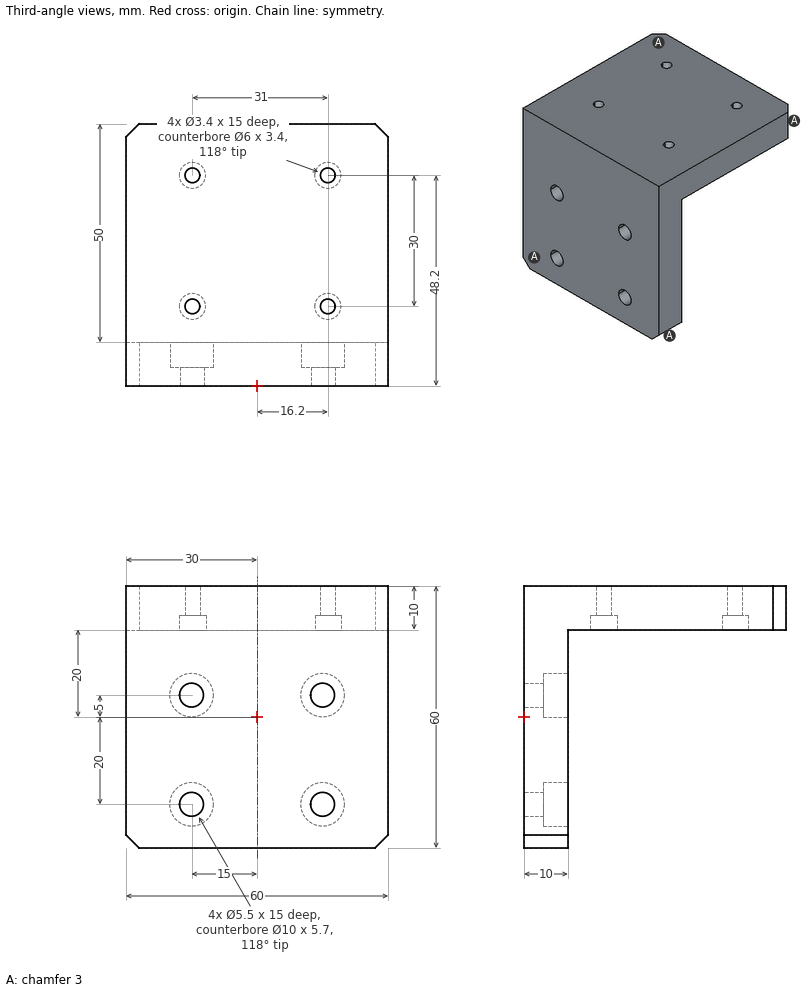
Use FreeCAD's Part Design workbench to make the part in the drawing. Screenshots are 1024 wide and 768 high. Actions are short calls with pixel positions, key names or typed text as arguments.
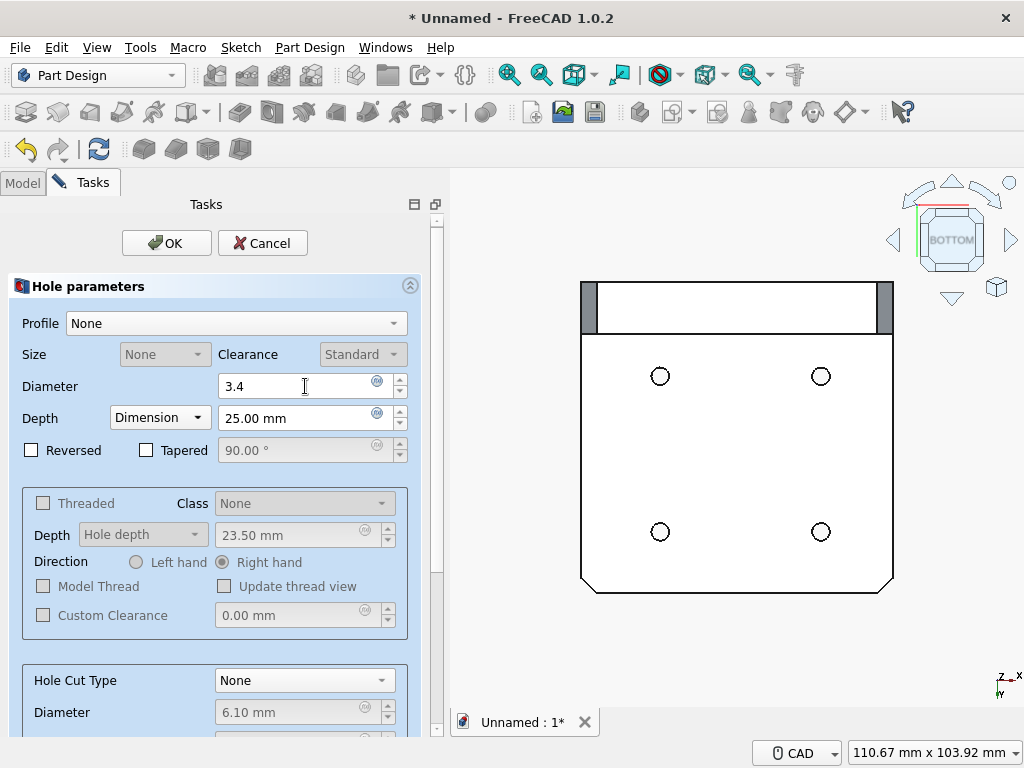
triple_click(305, 418)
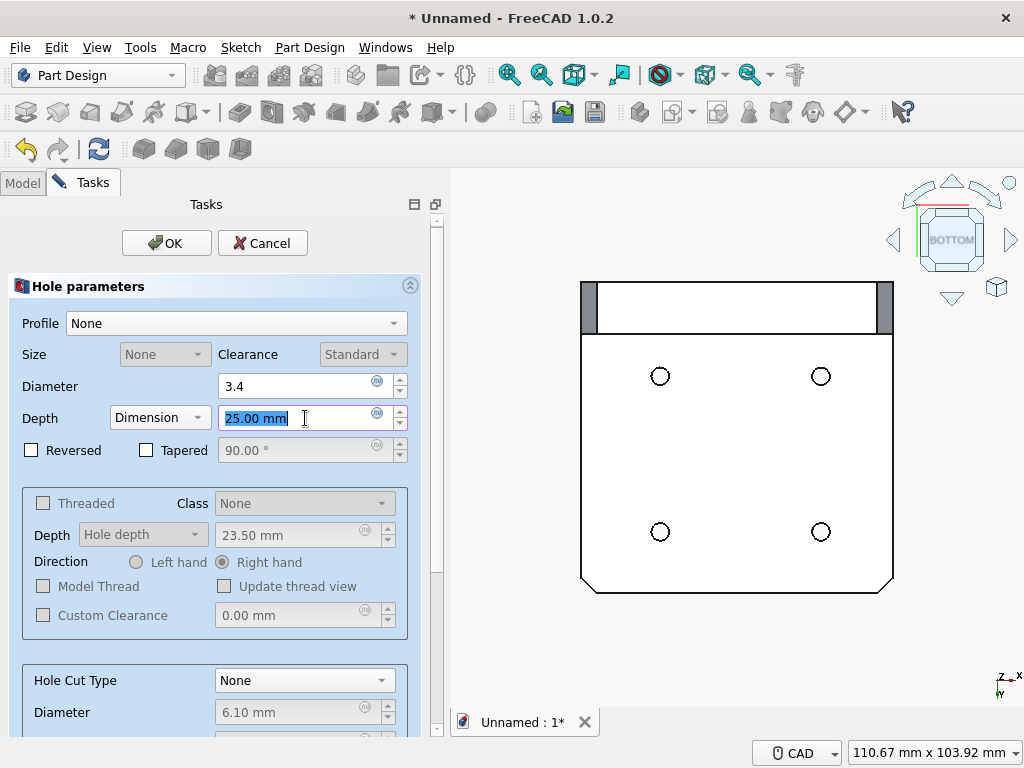
text(15)
key(Tab)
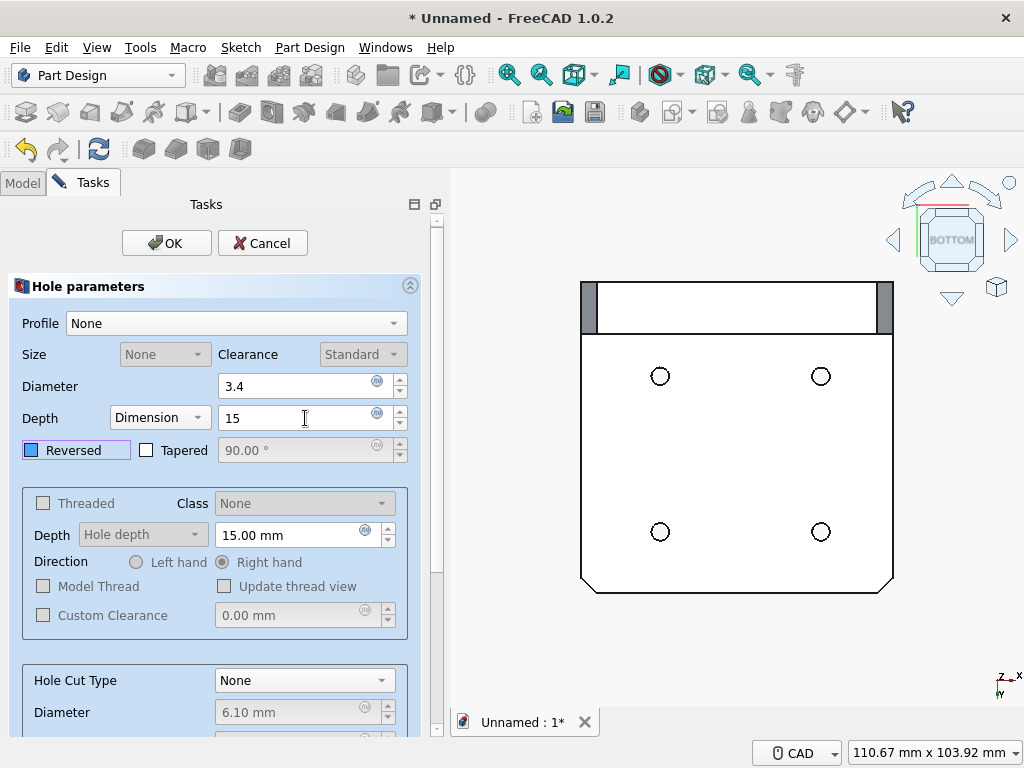
click(306, 680)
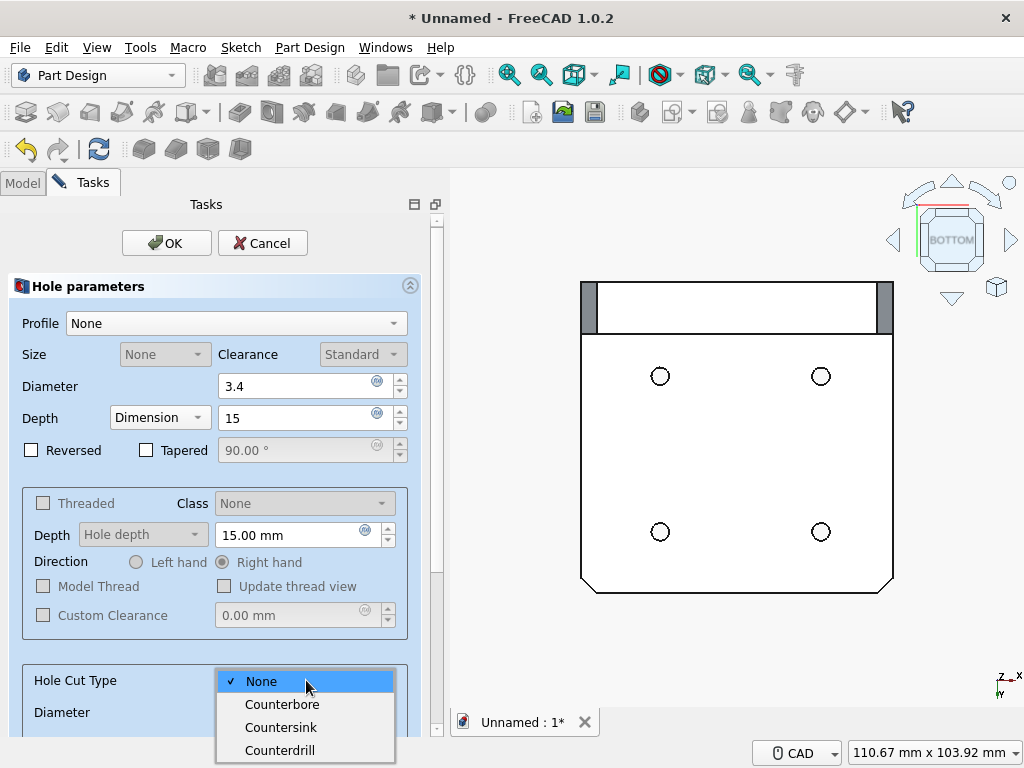
click(304, 704)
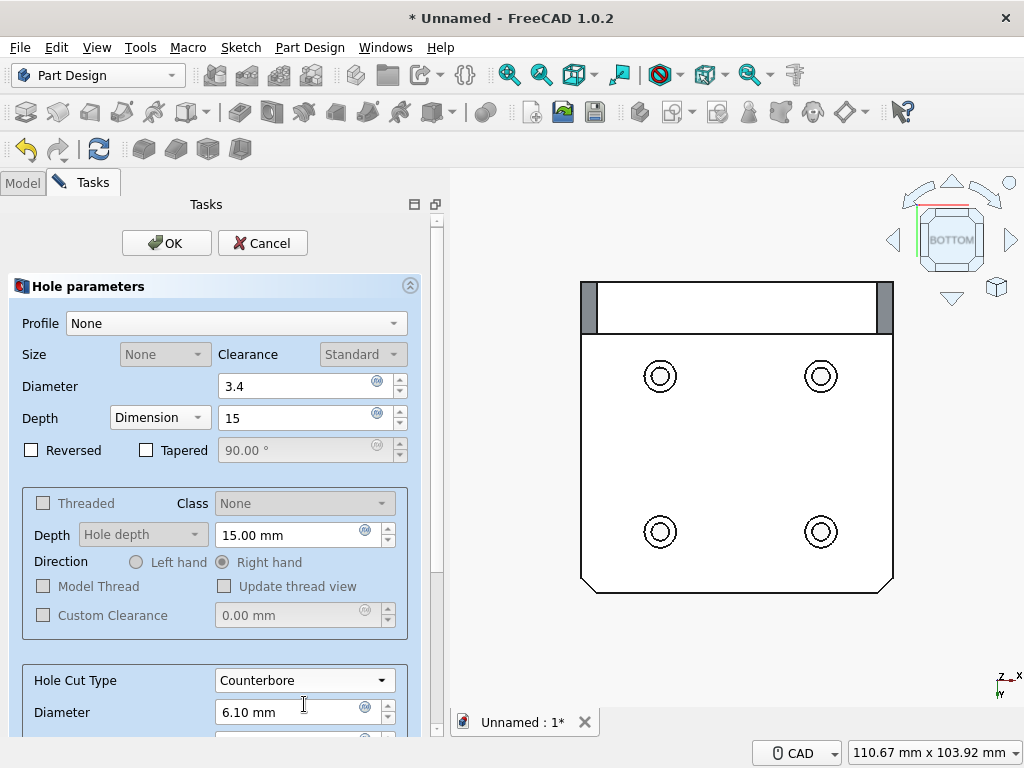
triple_click(298, 712)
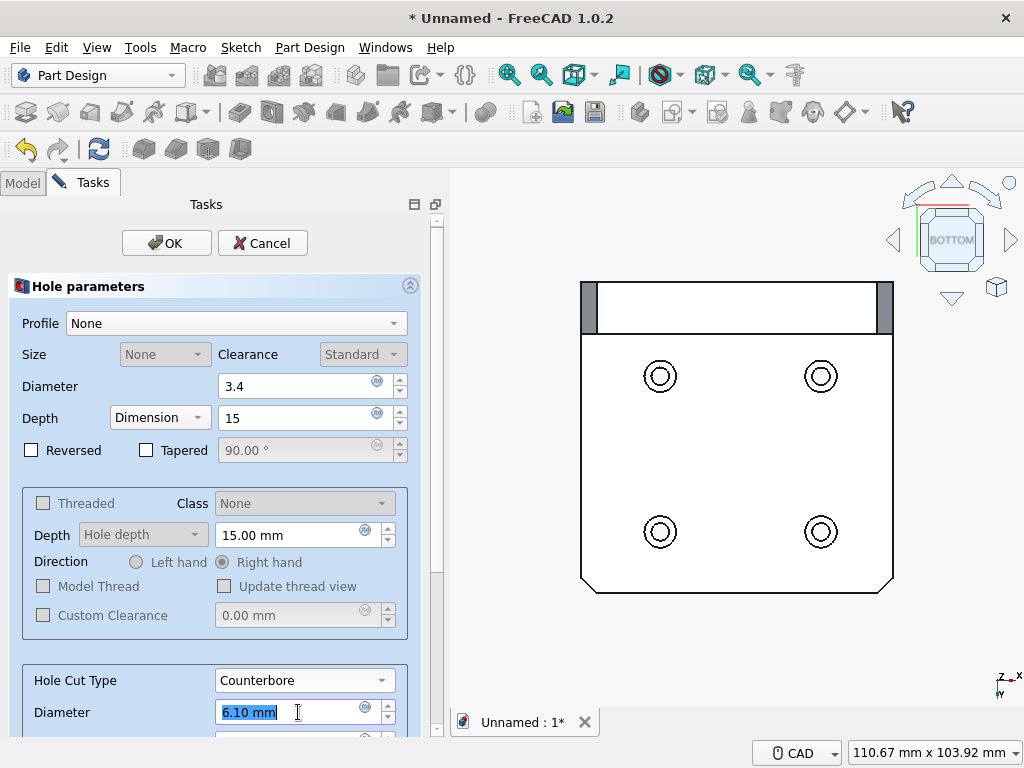
text(6)
key(Tab)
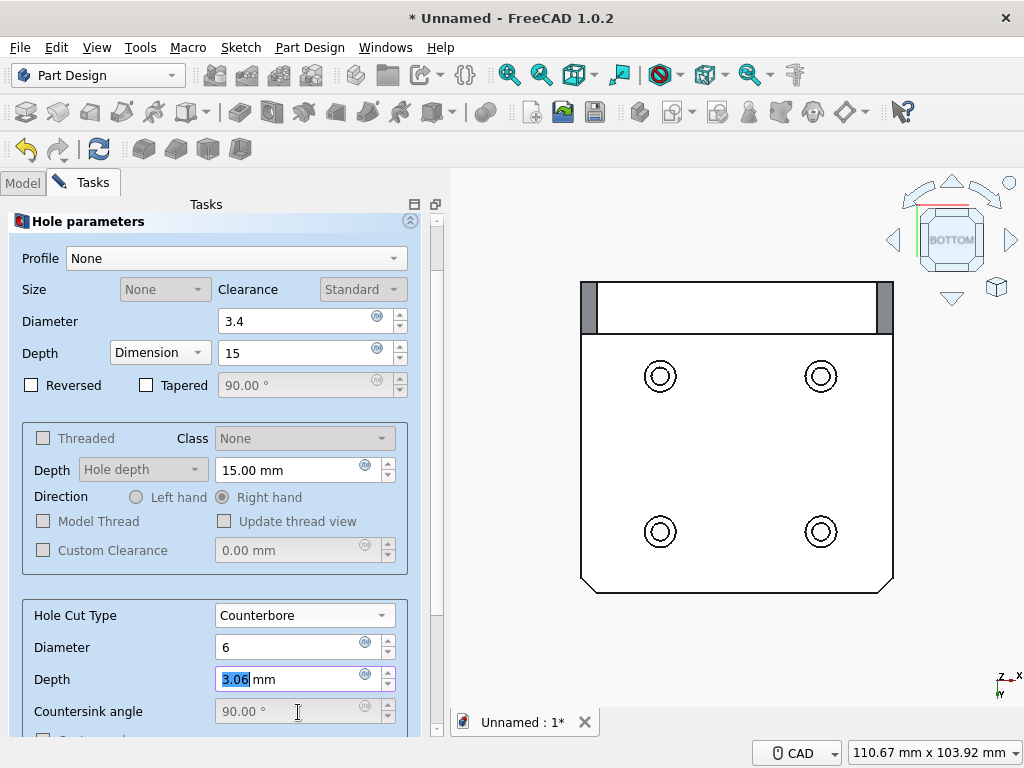
text(3.4)
key(Tab)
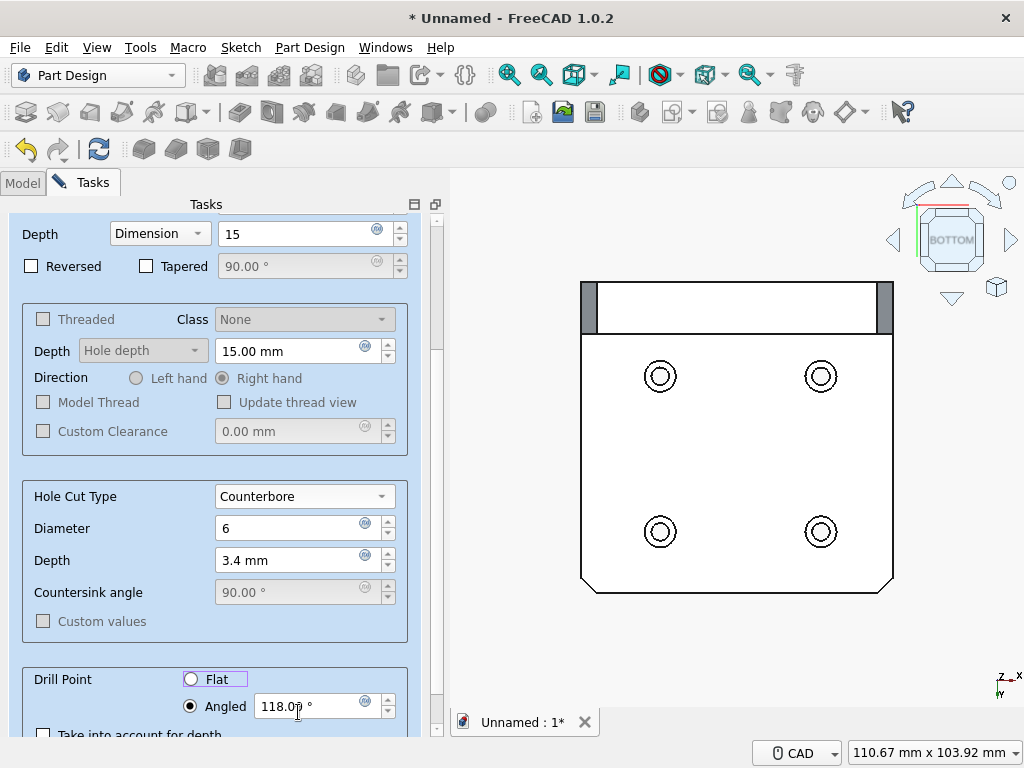
scroll(437, 475, up, 4)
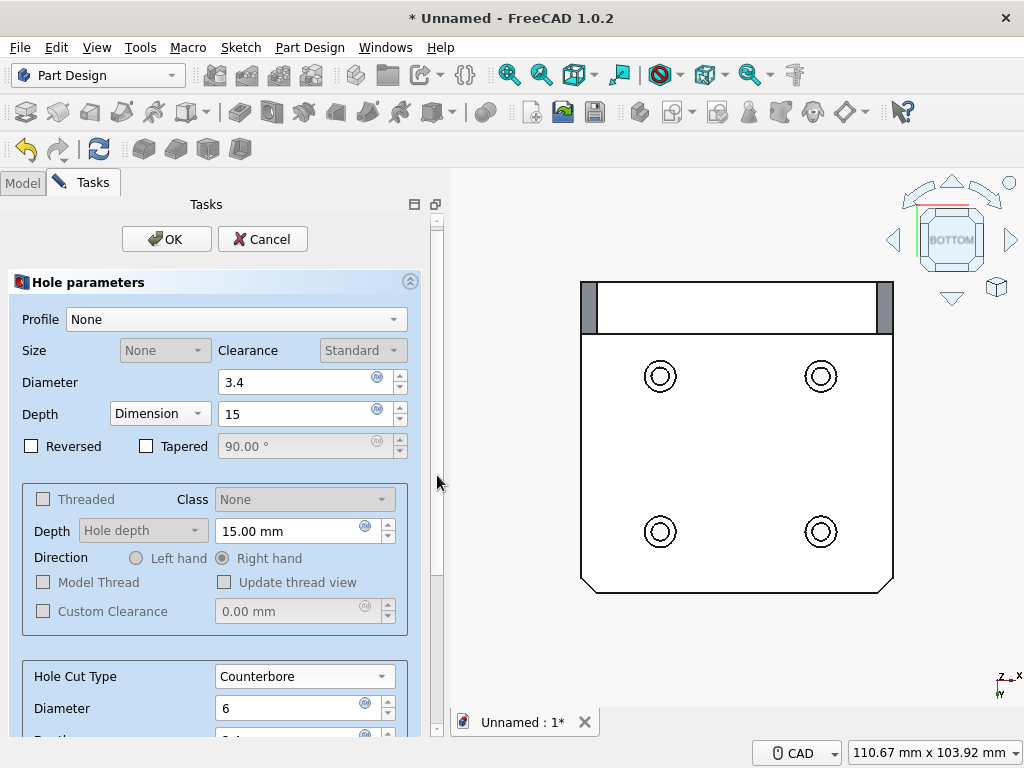
click(167, 243)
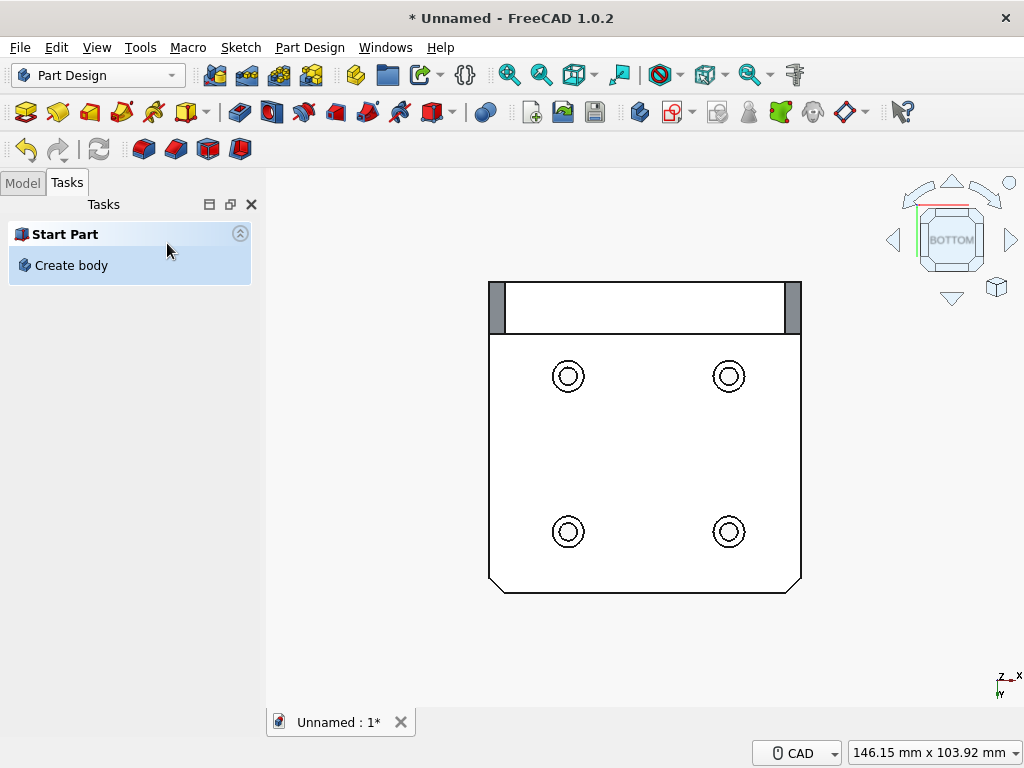
key(0)